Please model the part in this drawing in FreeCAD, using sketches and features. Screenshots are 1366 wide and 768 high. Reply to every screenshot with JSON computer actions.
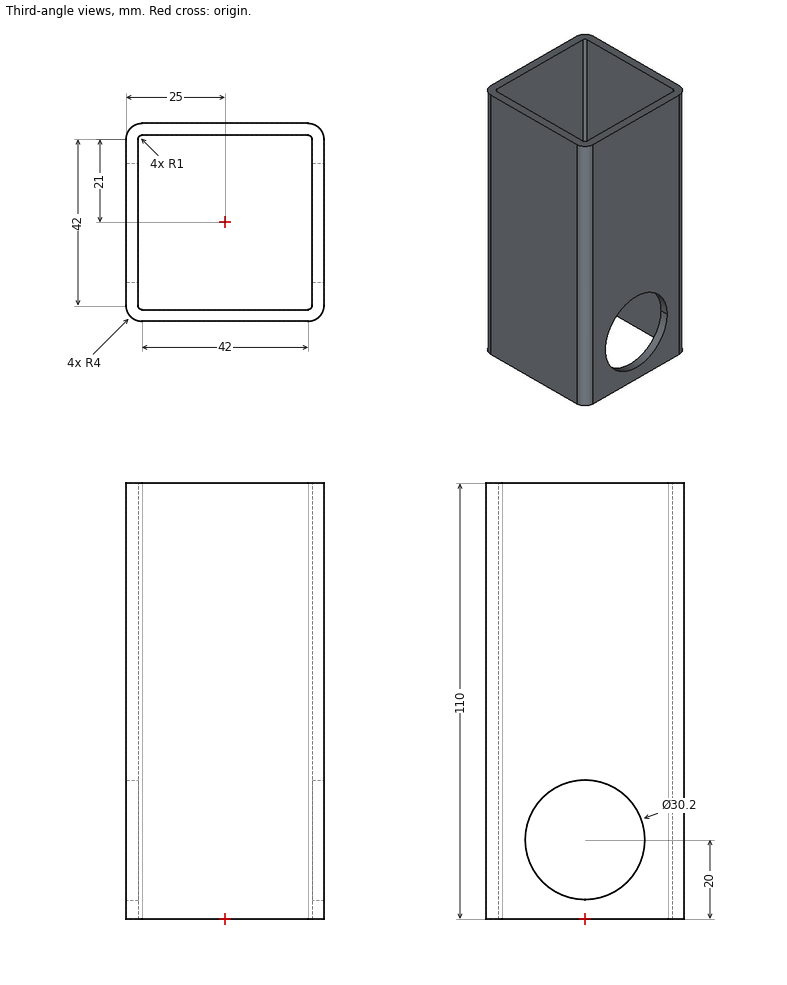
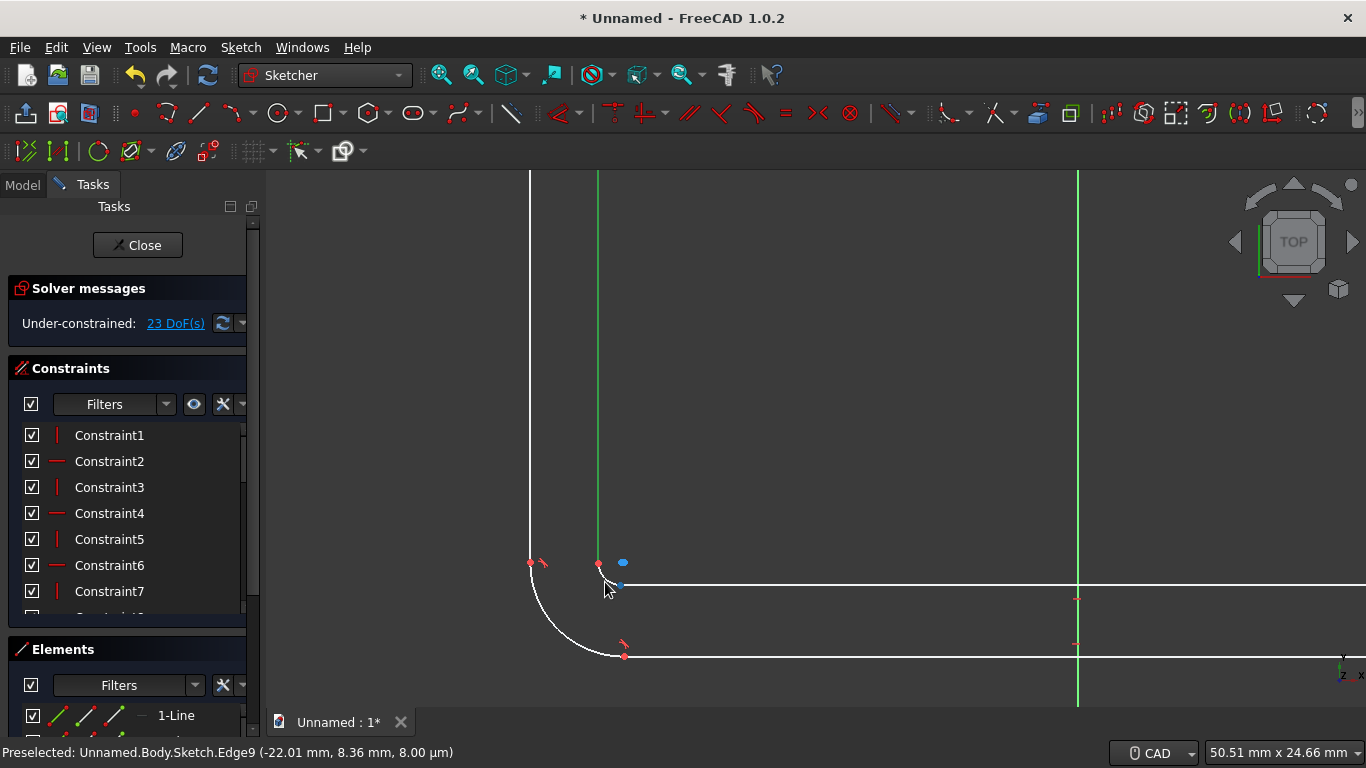
{"action": "left_click", "coordinate": [605, 579]}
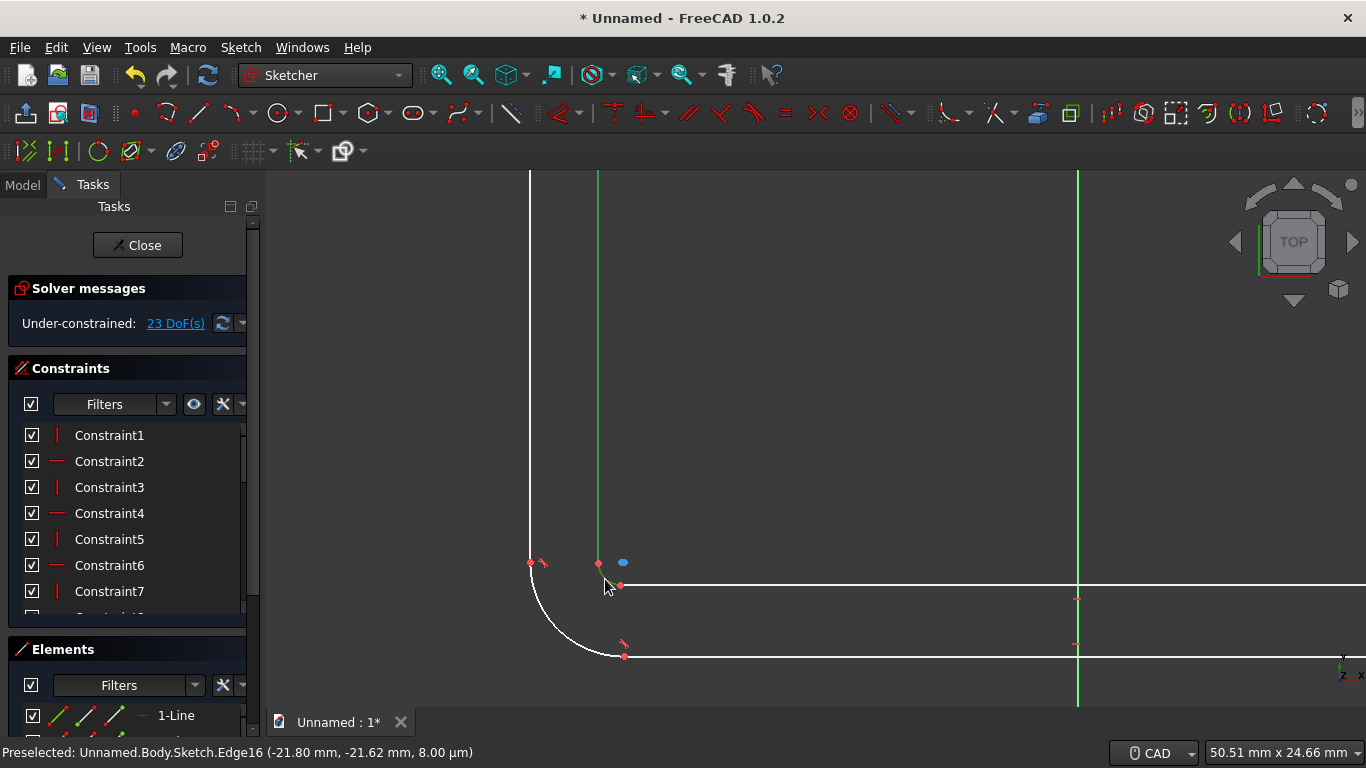
{"action": "left_click", "coordinate": [754, 114]}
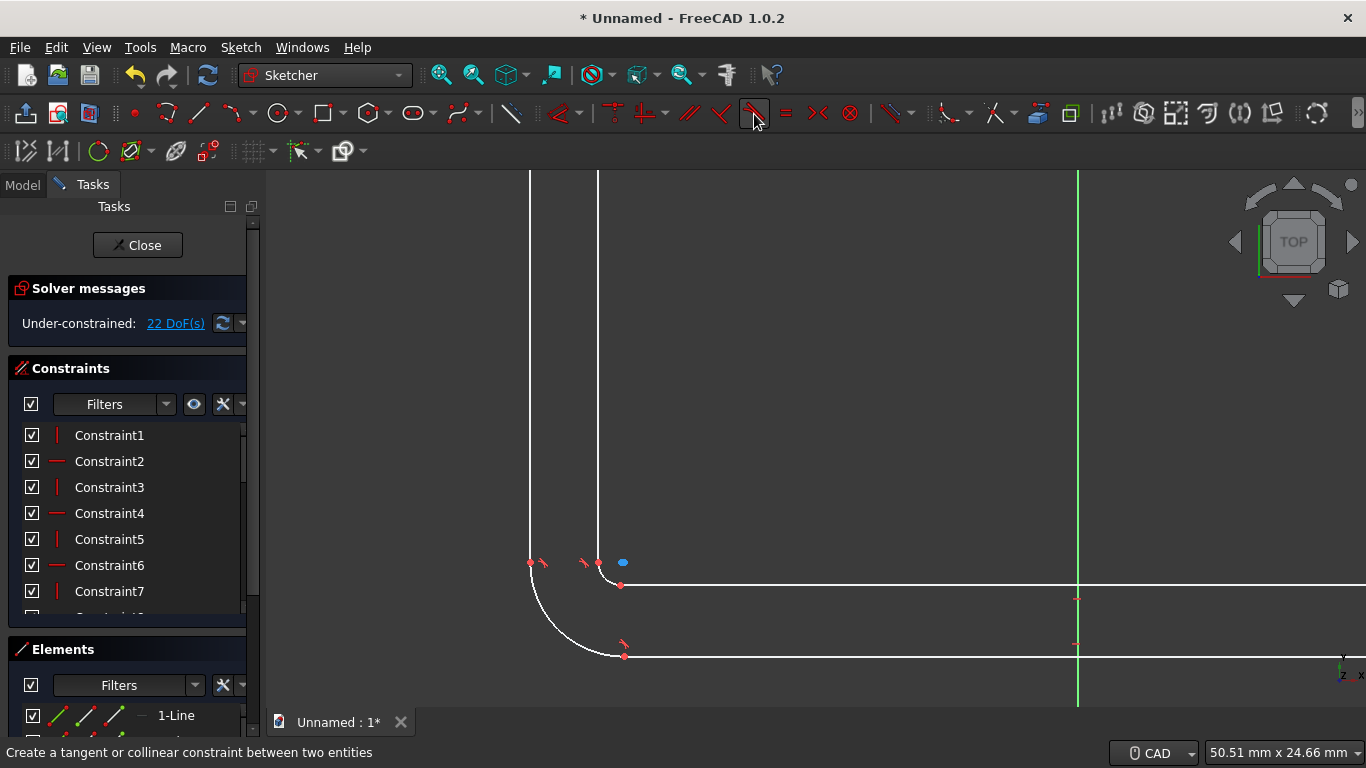
{"action": "scroll", "coordinate": [605, 582], "scroll_direction": "down", "scroll_amount": 6}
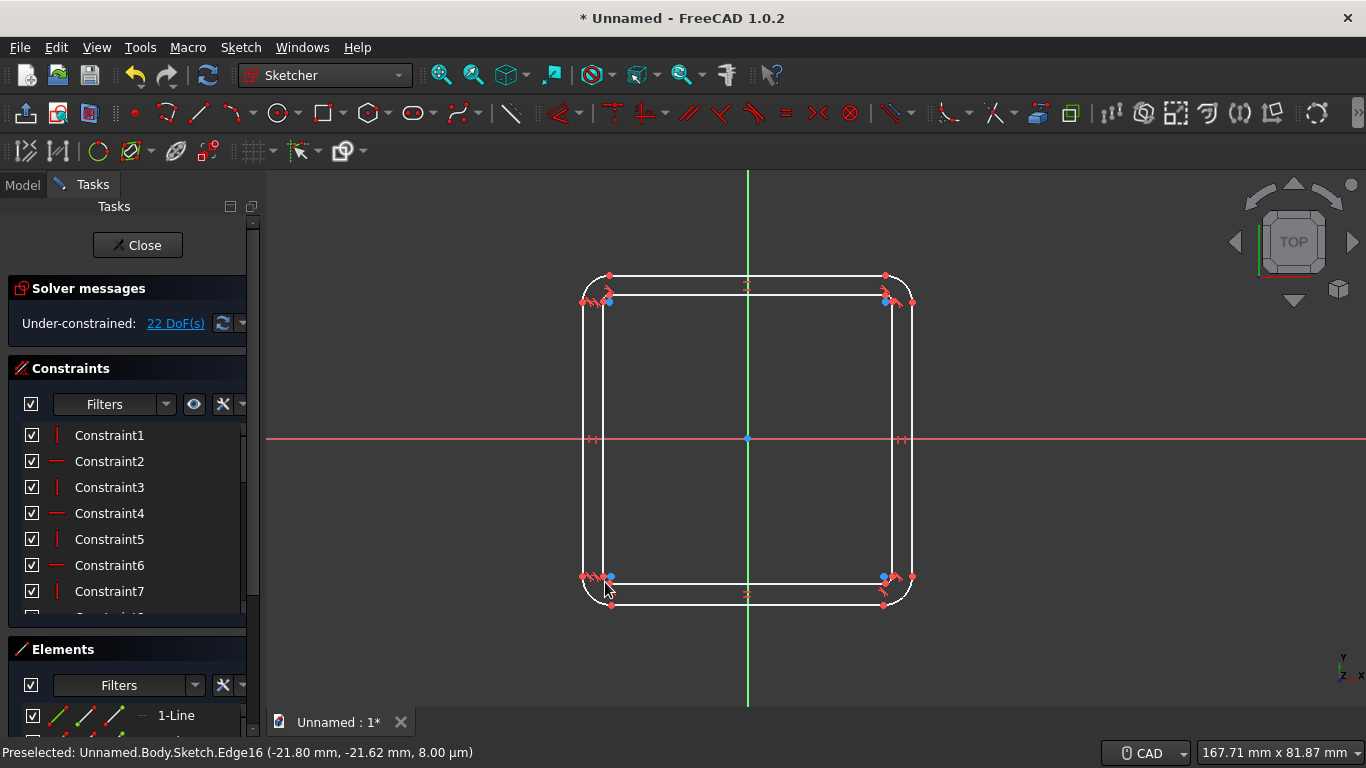
{"action": "left_click", "coordinate": [693, 295]}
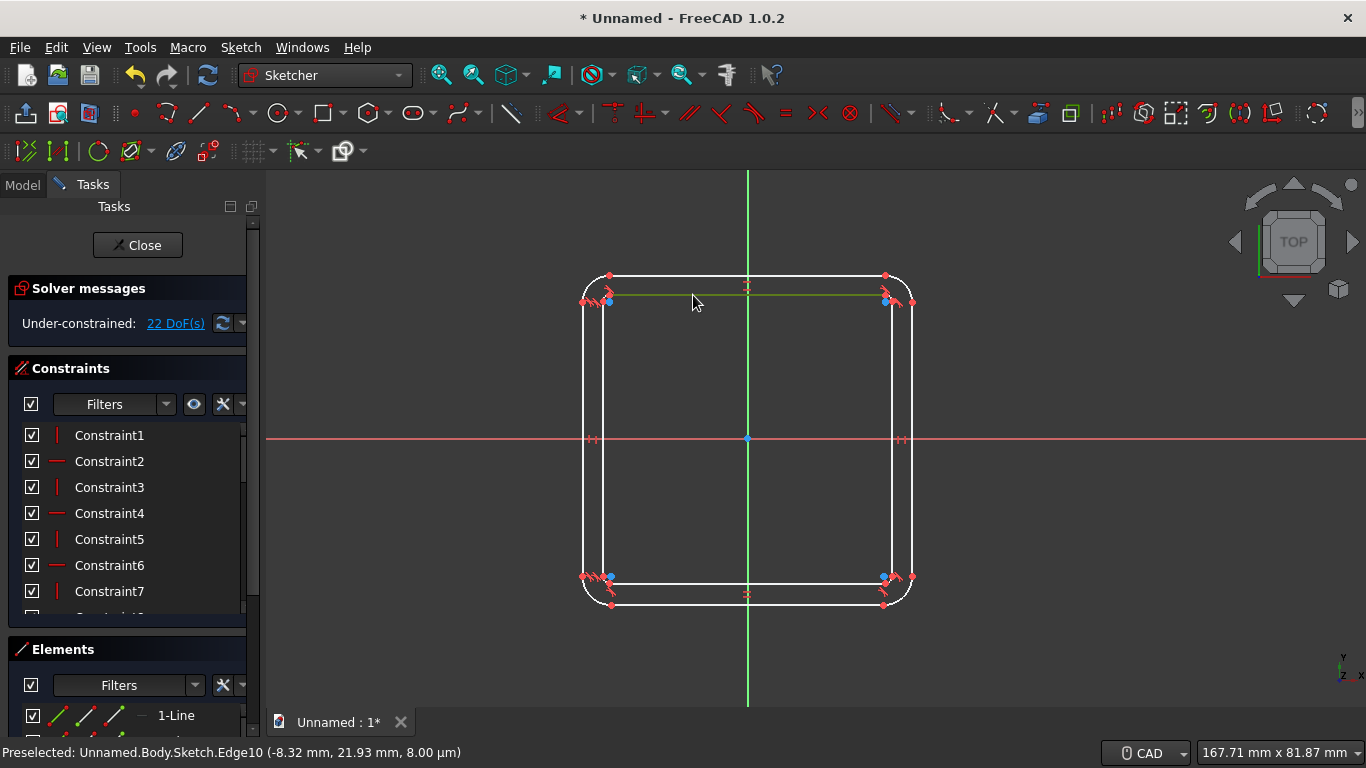
{"action": "scroll", "coordinate": [605, 297], "scroll_direction": "up", "scroll_amount": 6}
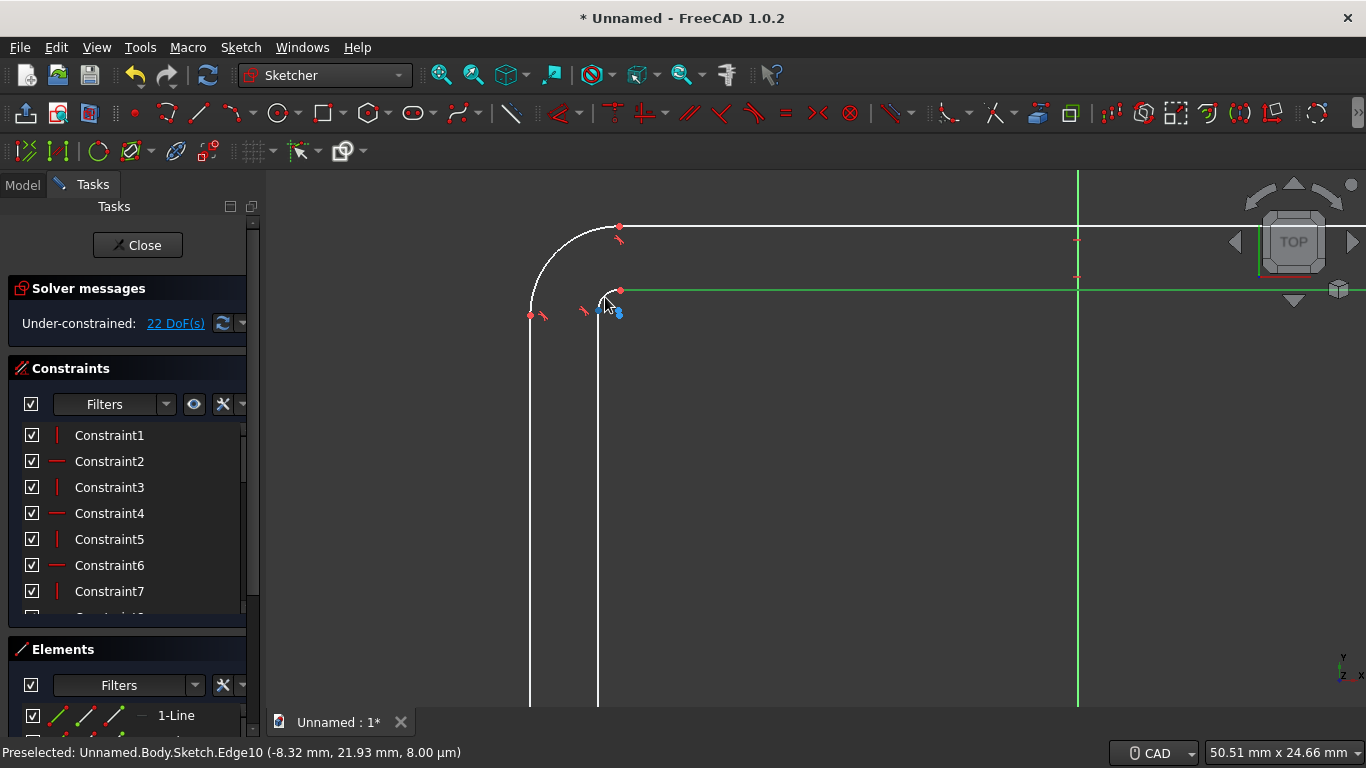
{"action": "left_click", "coordinate": [605, 295]}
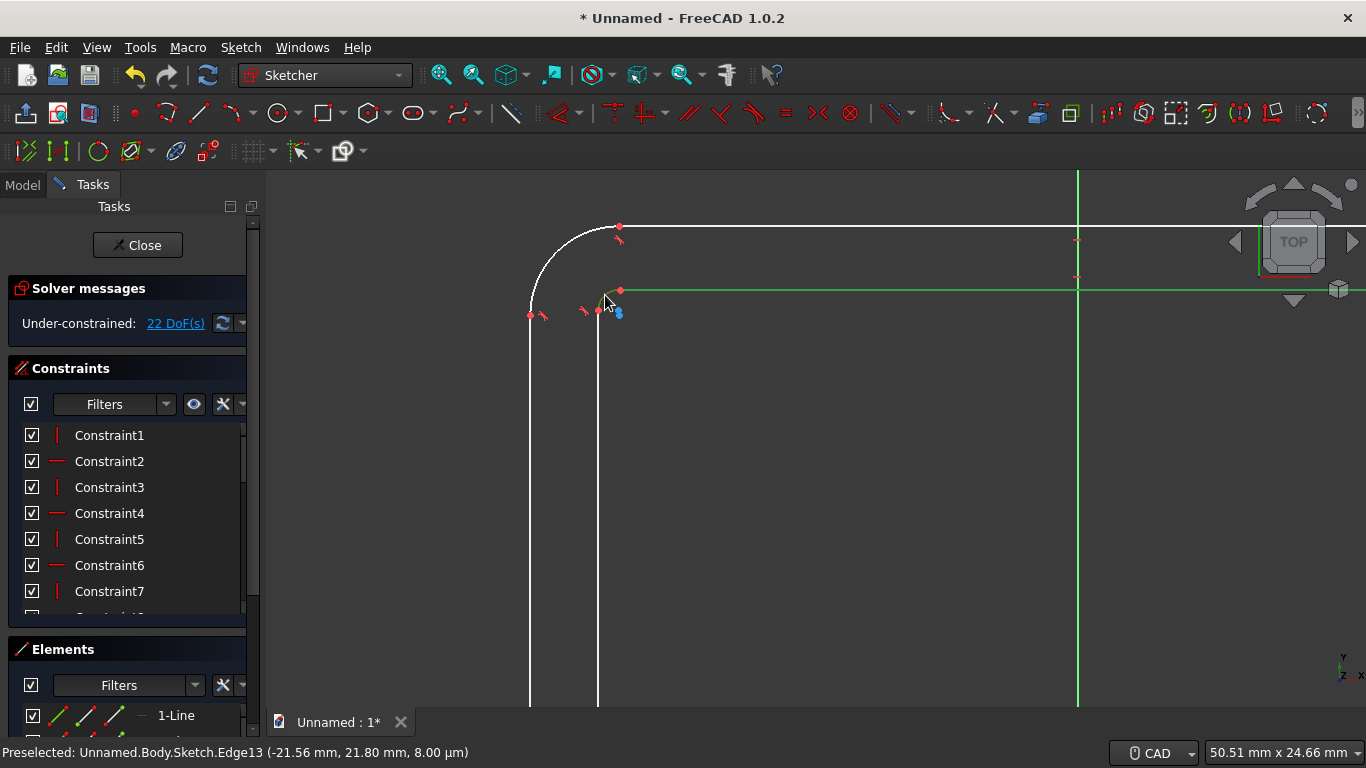
{"action": "left_click", "coordinate": [754, 114]}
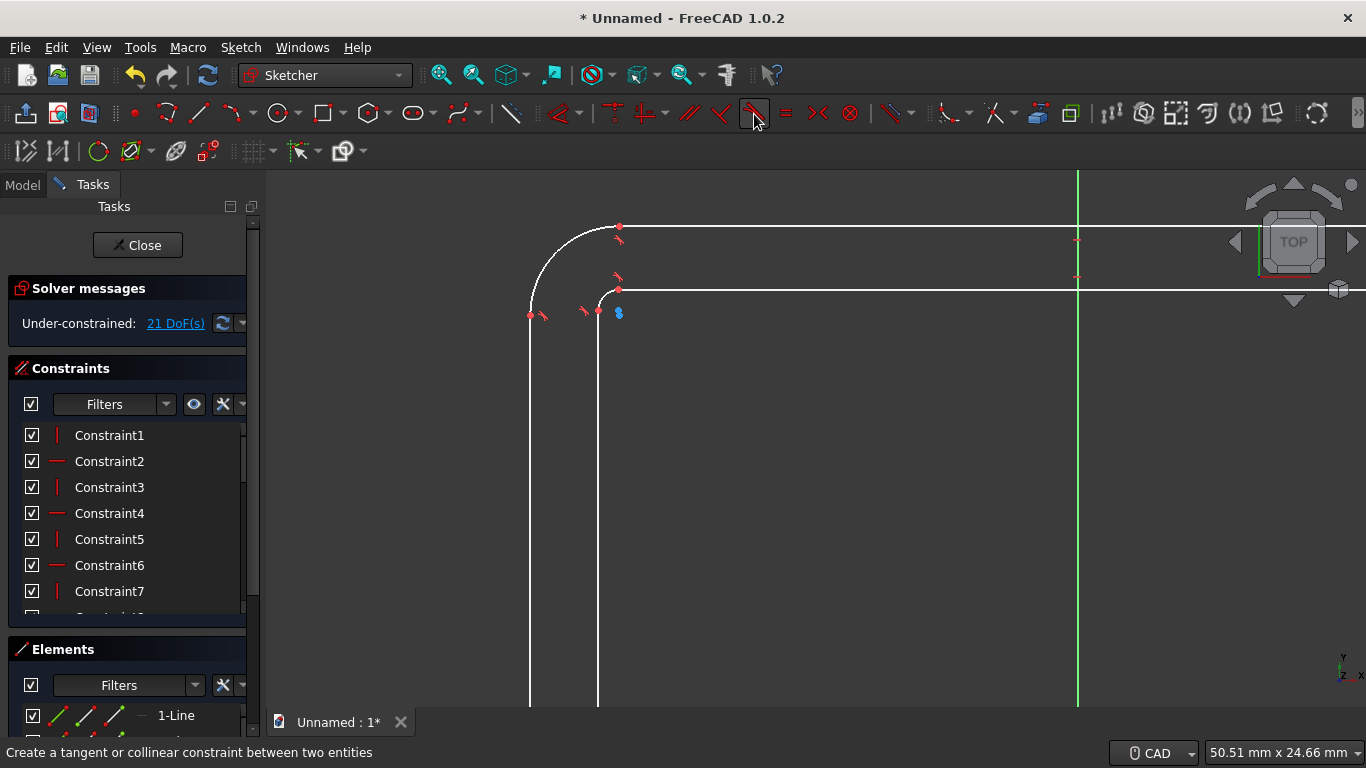
{"action": "scroll", "coordinate": [605, 297], "scroll_direction": "down", "scroll_amount": 6}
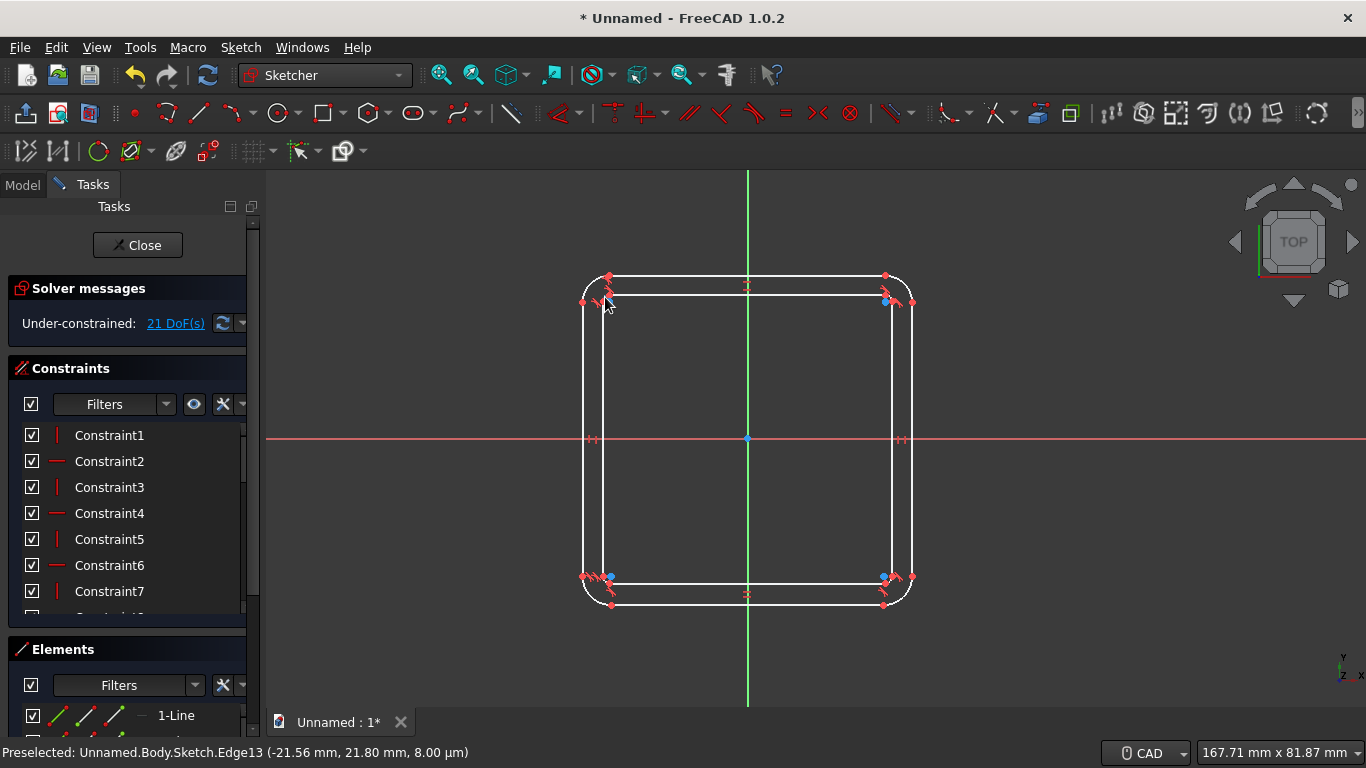
{"action": "left_click", "coordinate": [692, 295]}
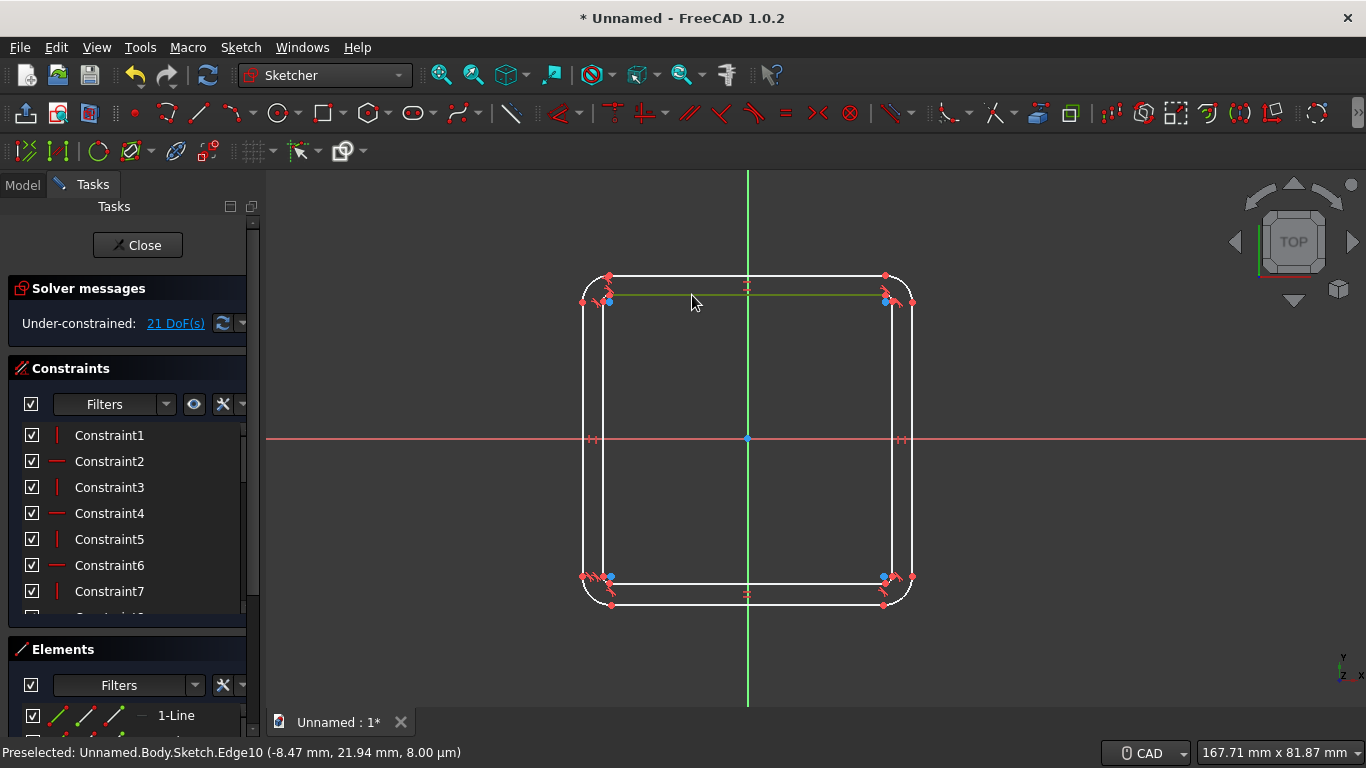
{"action": "scroll", "coordinate": [890, 297], "scroll_direction": "up", "scroll_amount": 5}